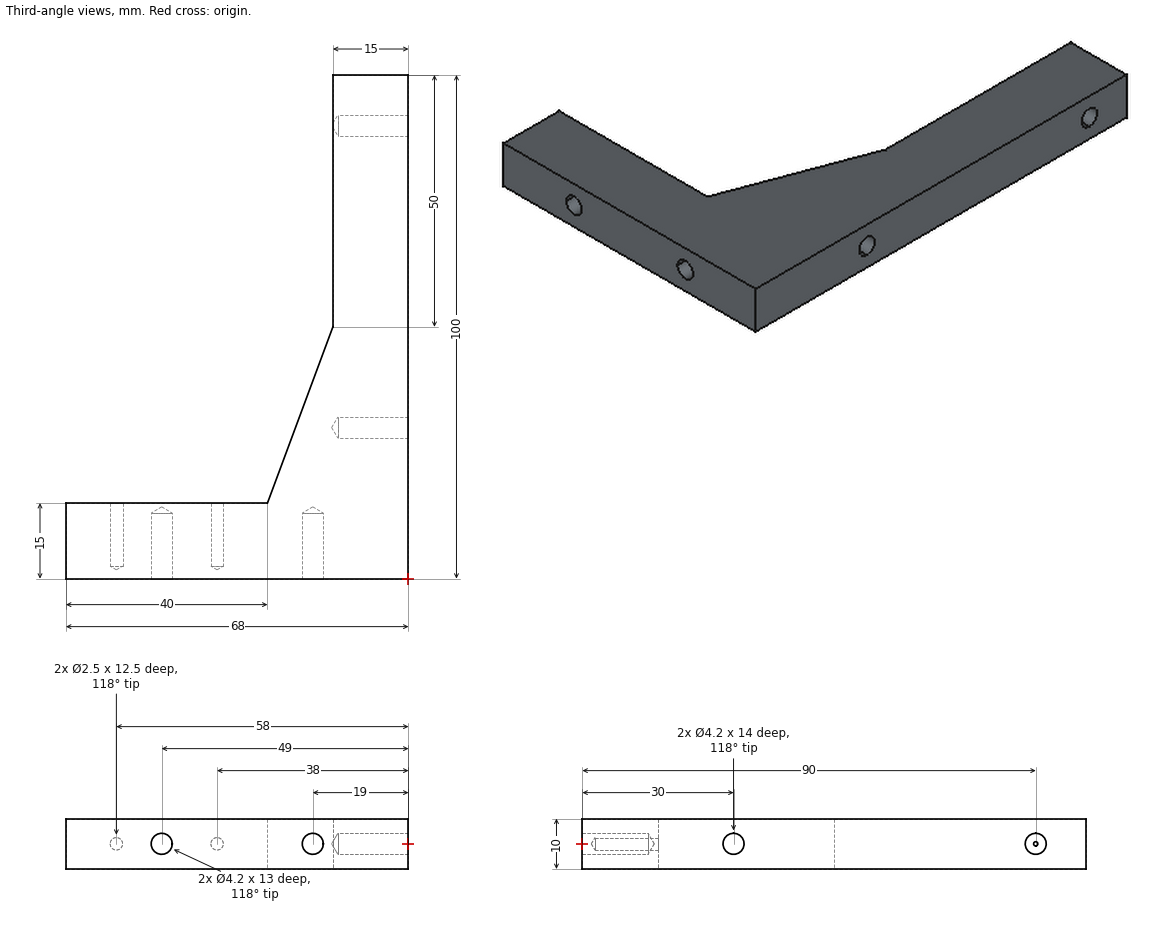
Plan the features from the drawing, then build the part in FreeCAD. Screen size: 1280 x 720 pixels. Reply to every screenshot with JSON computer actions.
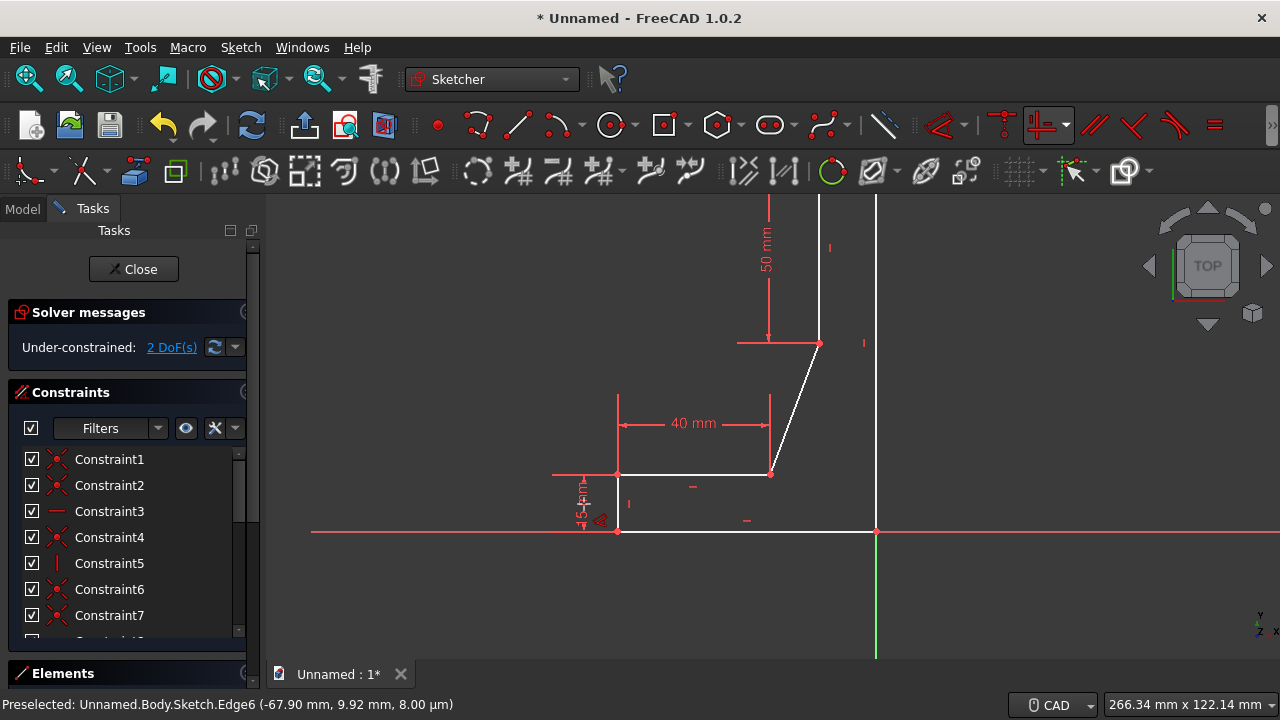
{"action": "left_click", "coordinate": [695, 532]}
{"action": "left_click", "coordinate": [747, 566]}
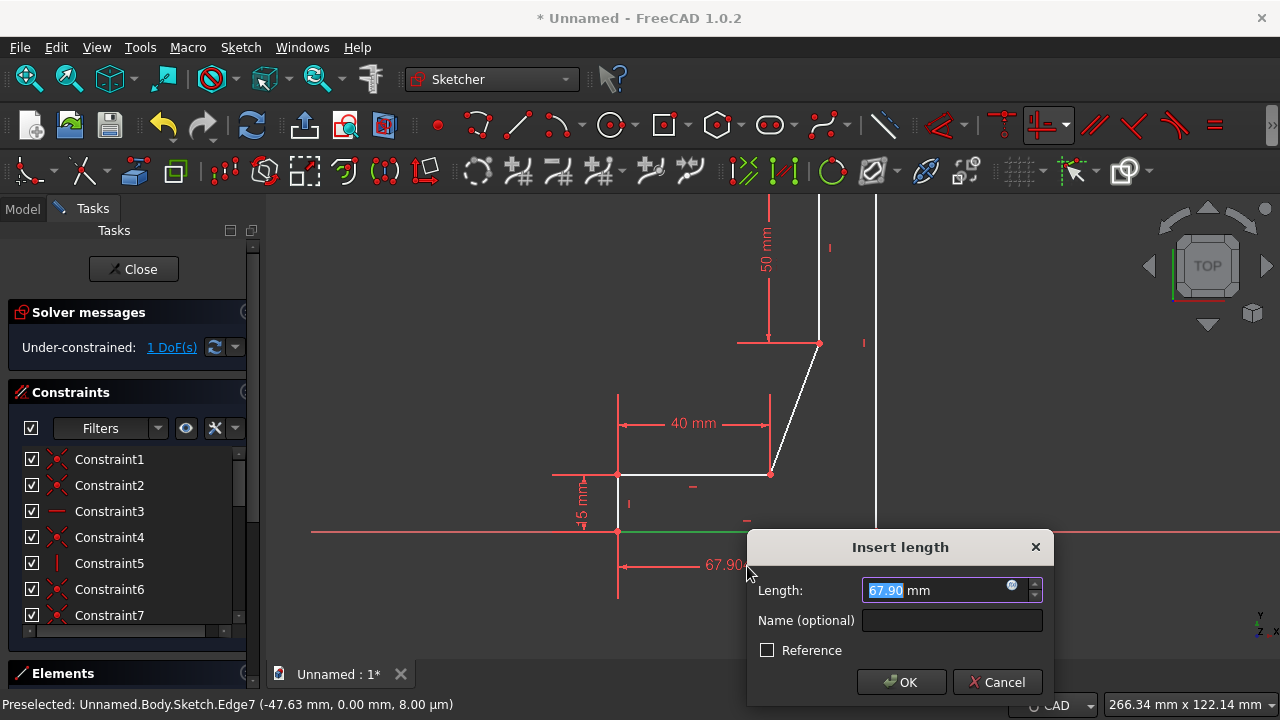
{"action": "type", "text": "68"}
{"action": "key", "text": "Return"}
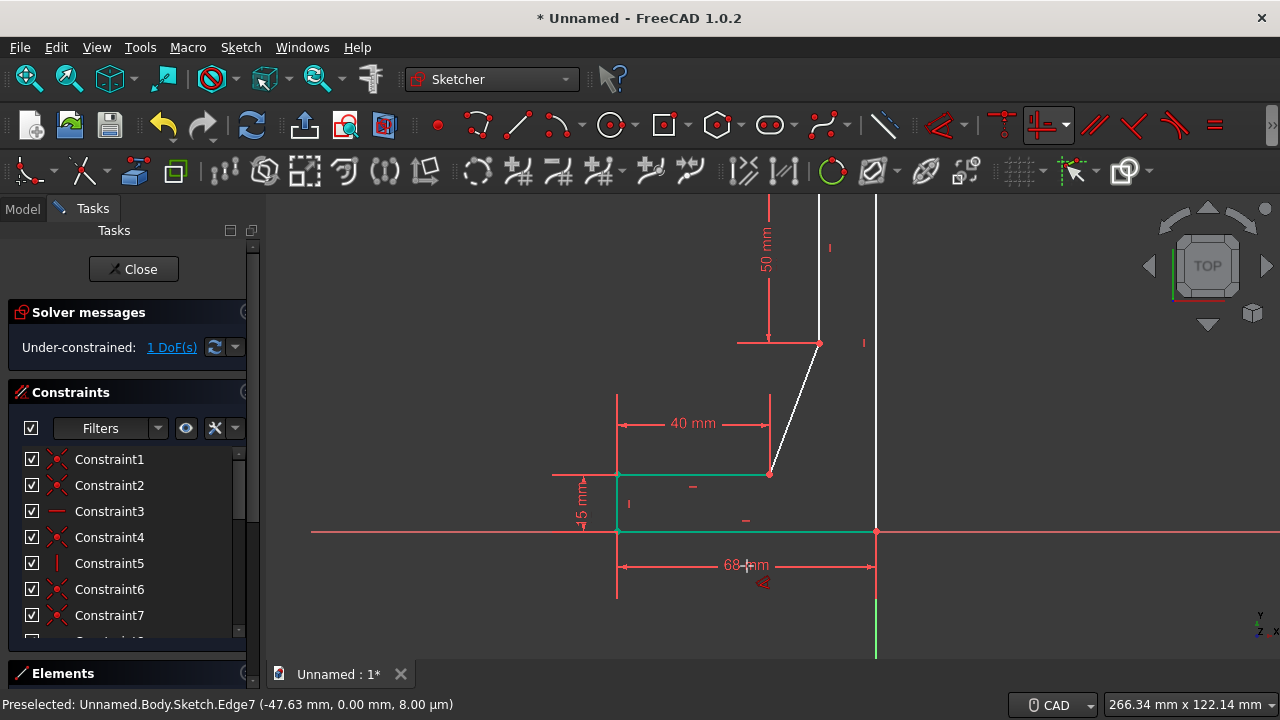
{"action": "left_click", "coordinate": [876, 418]}
{"action": "left_click", "coordinate": [910, 377]}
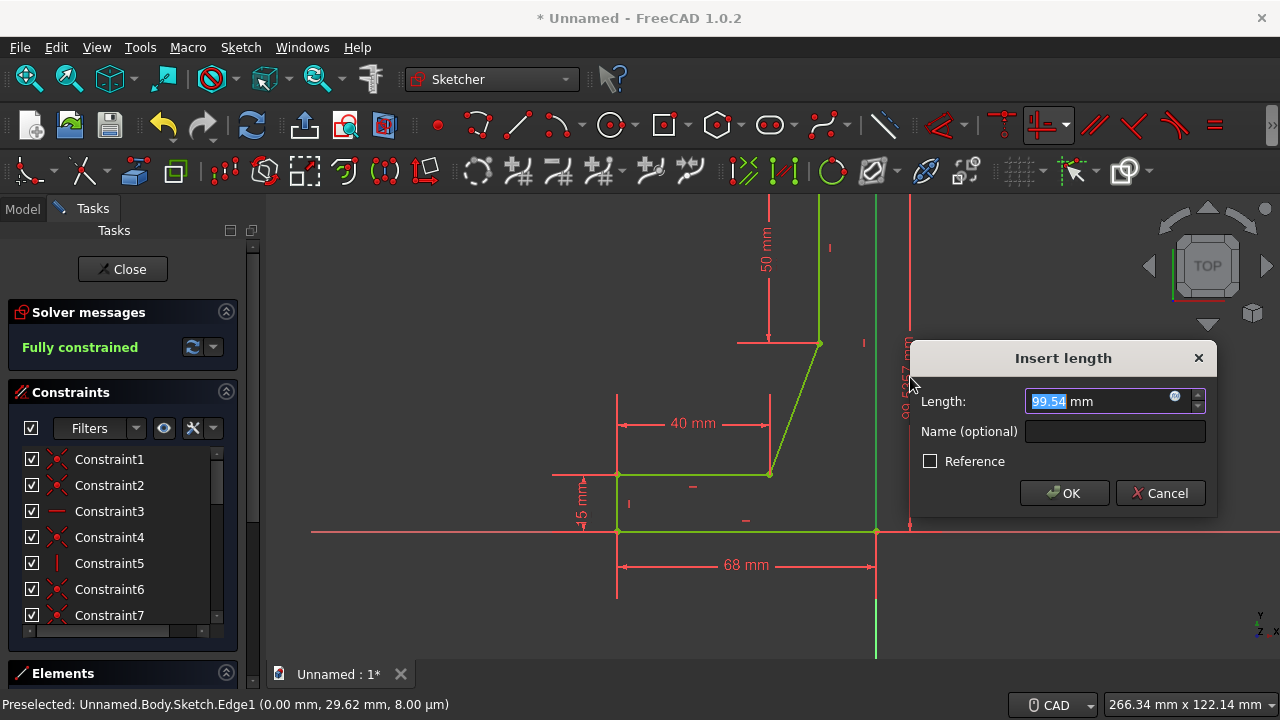
{"action": "type", "text": "100"}
{"action": "key", "text": "Return"}
{"action": "key", "text": "Escape"}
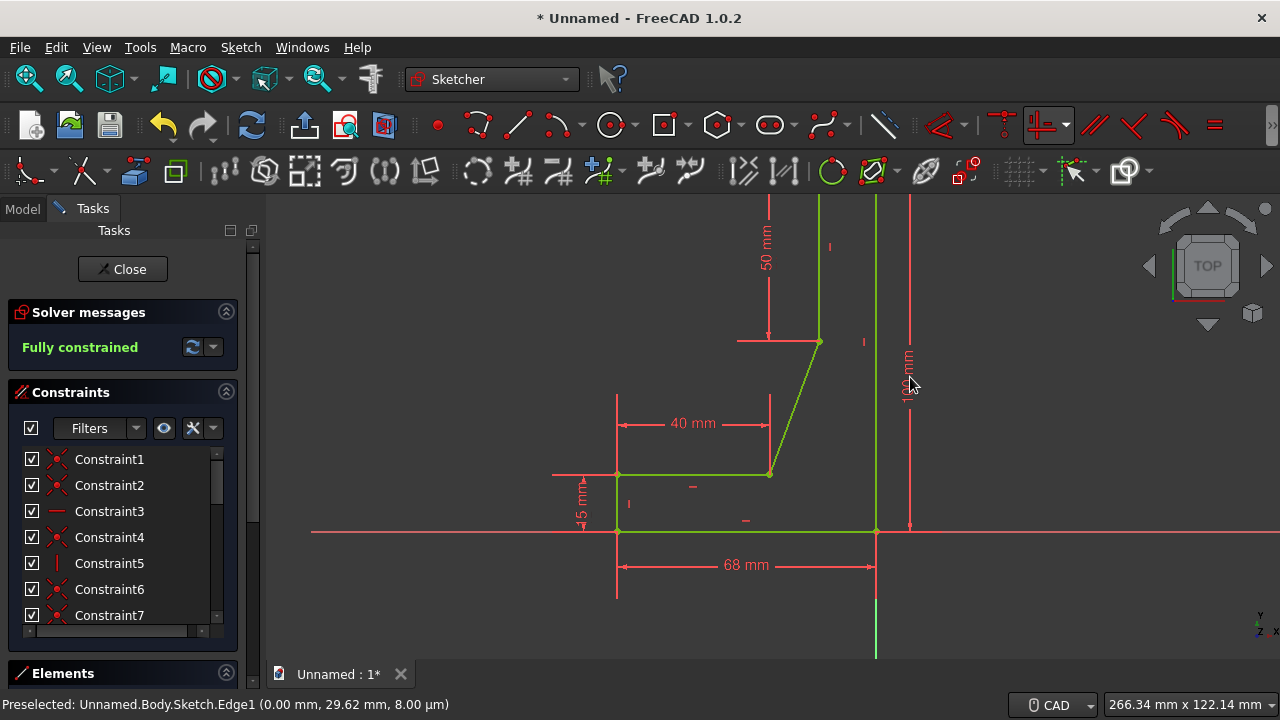
{"action": "left_click", "coordinate": [123, 269]}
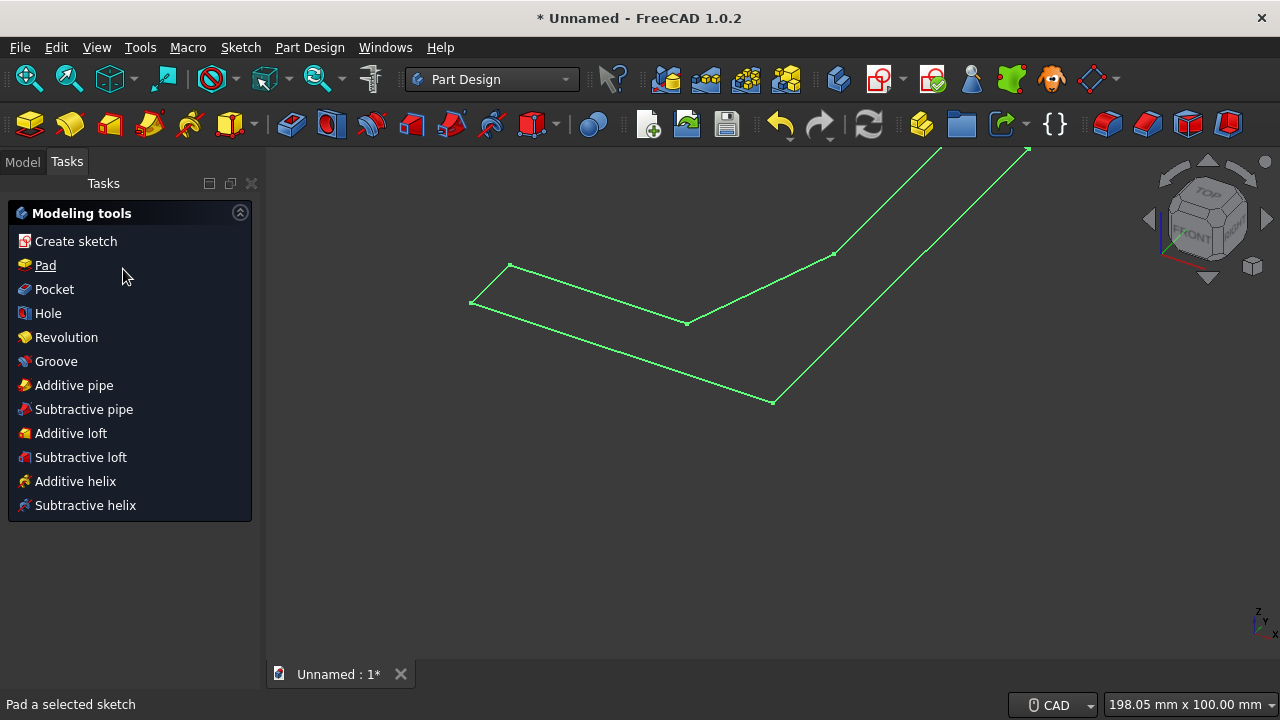
{"action": "left_click", "coordinate": [30, 124]}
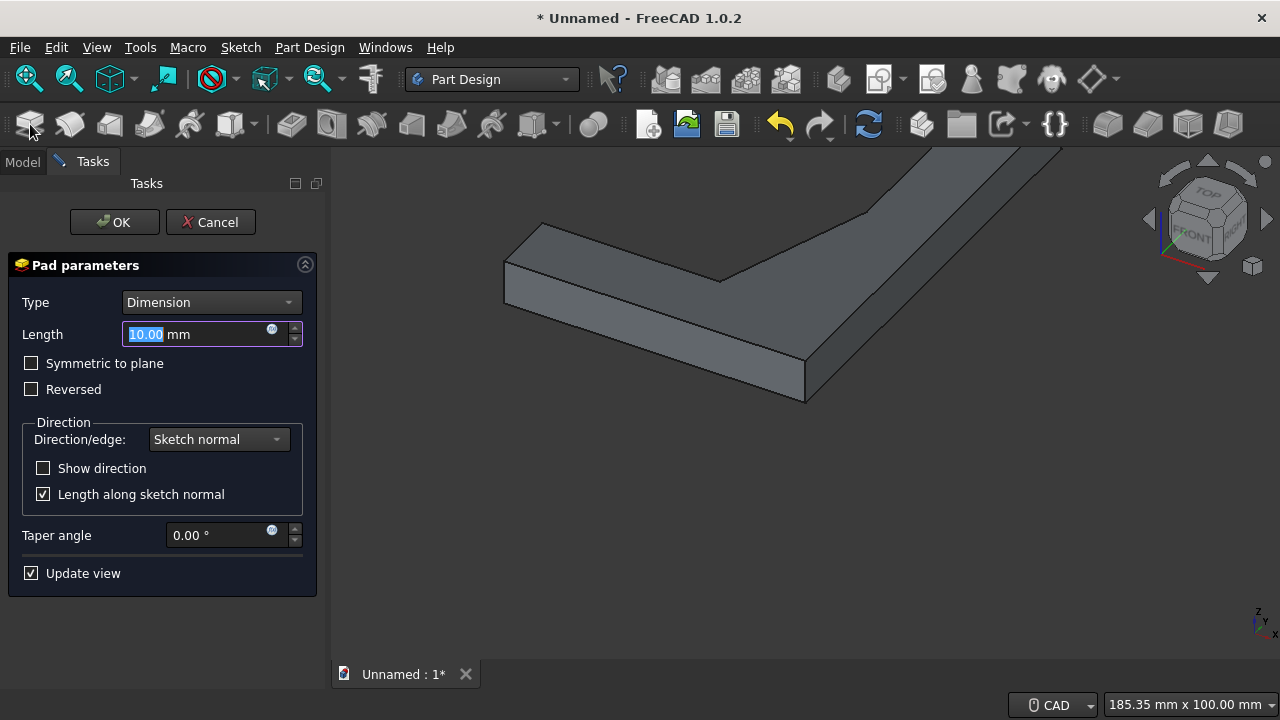
{"action": "type", "text": "10"}
{"action": "key", "text": "Tab"}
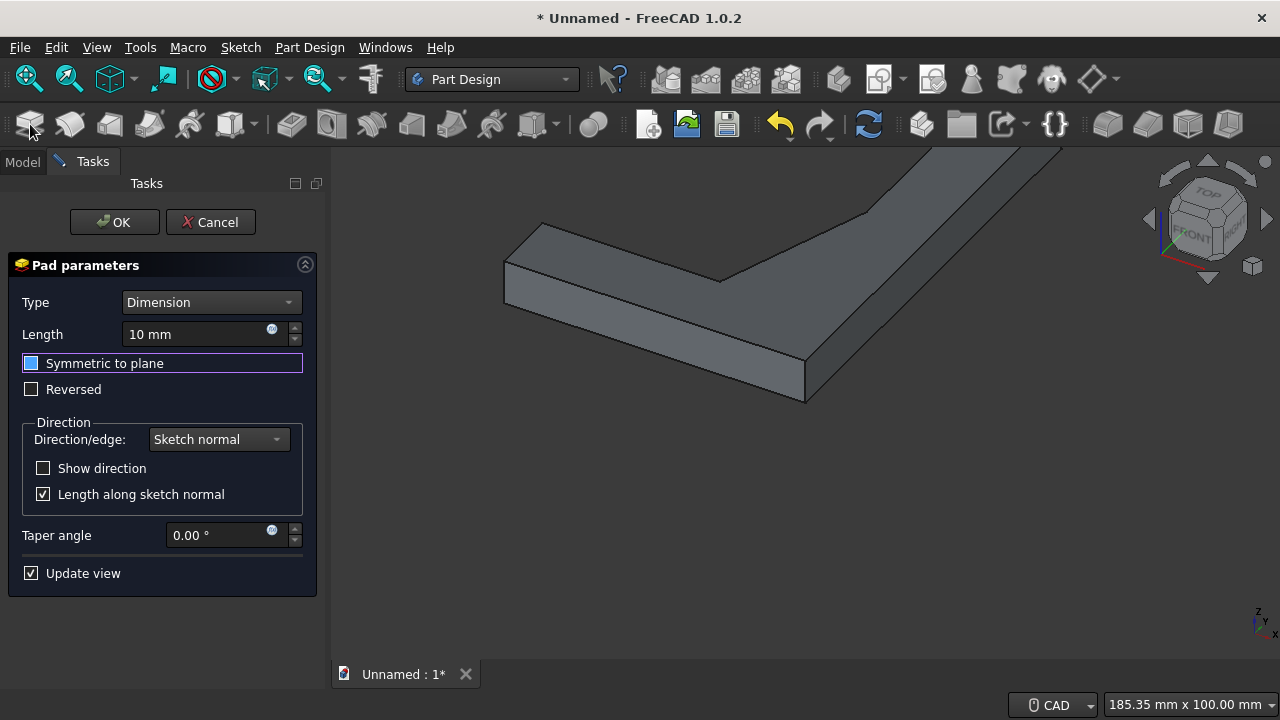
{"action": "left_click", "coordinate": [30, 363]}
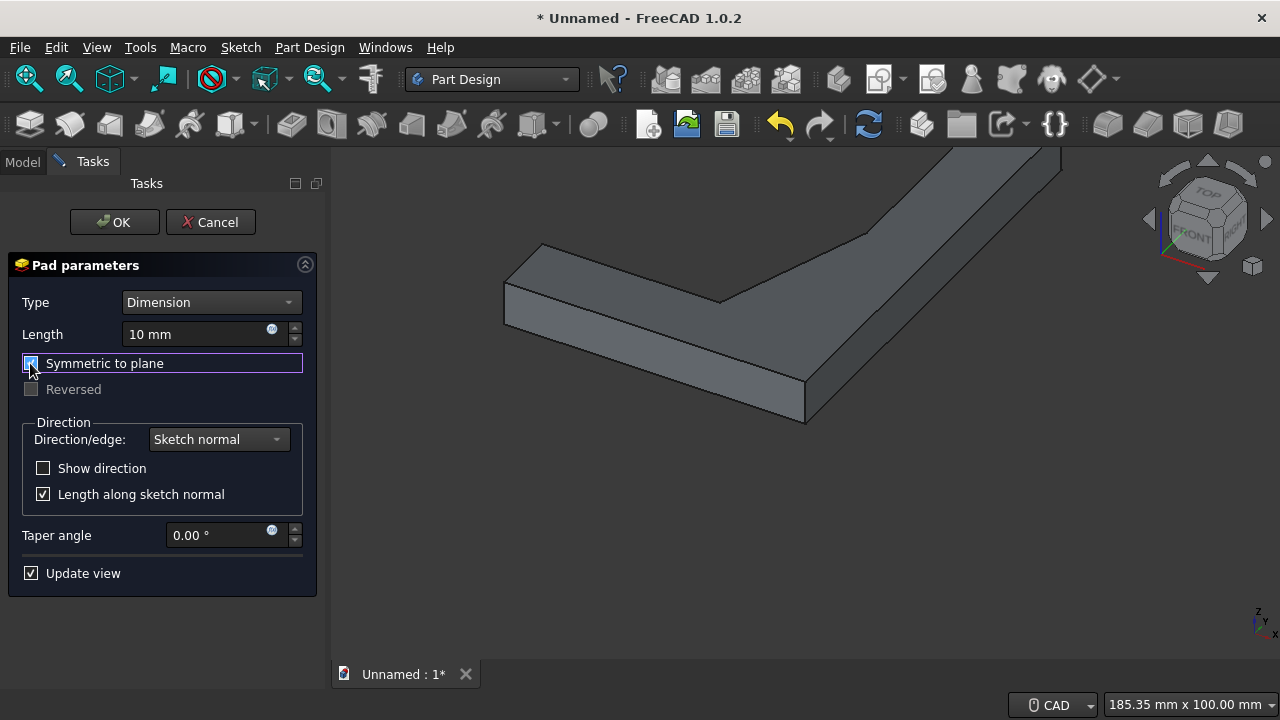
{"action": "left_click", "coordinate": [115, 222]}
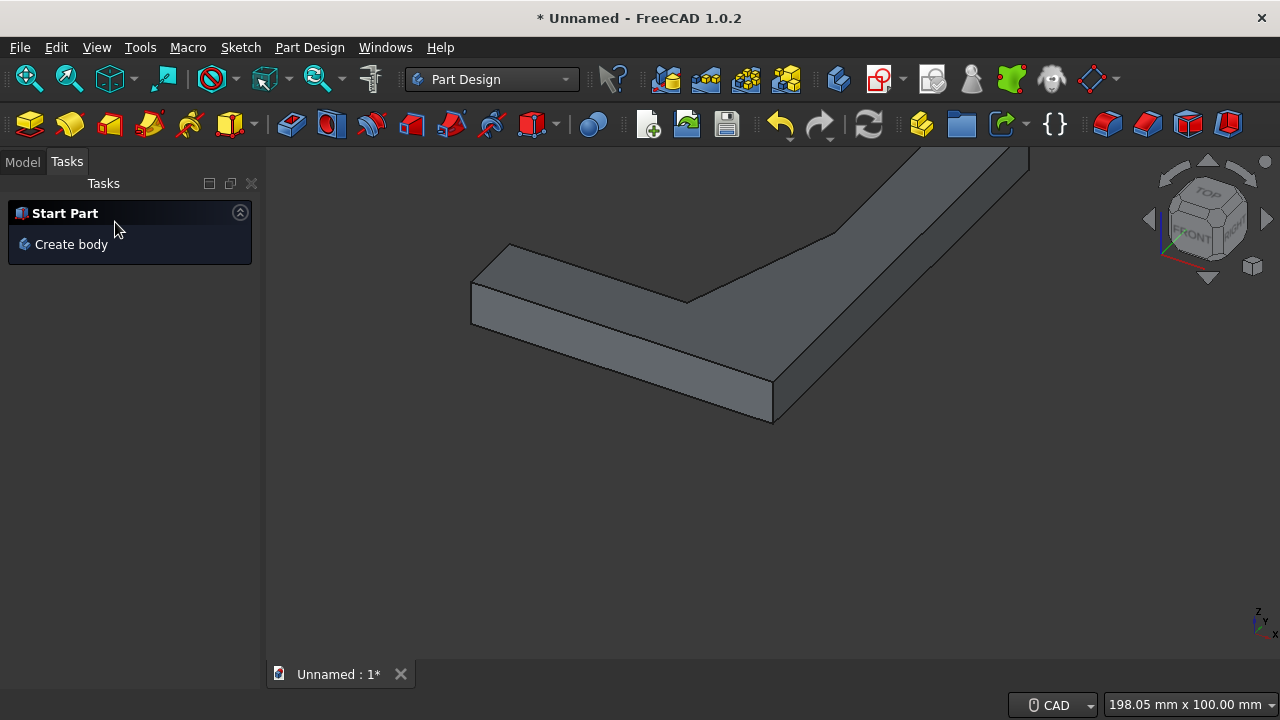
{"action": "left_click", "coordinate": [30, 80]}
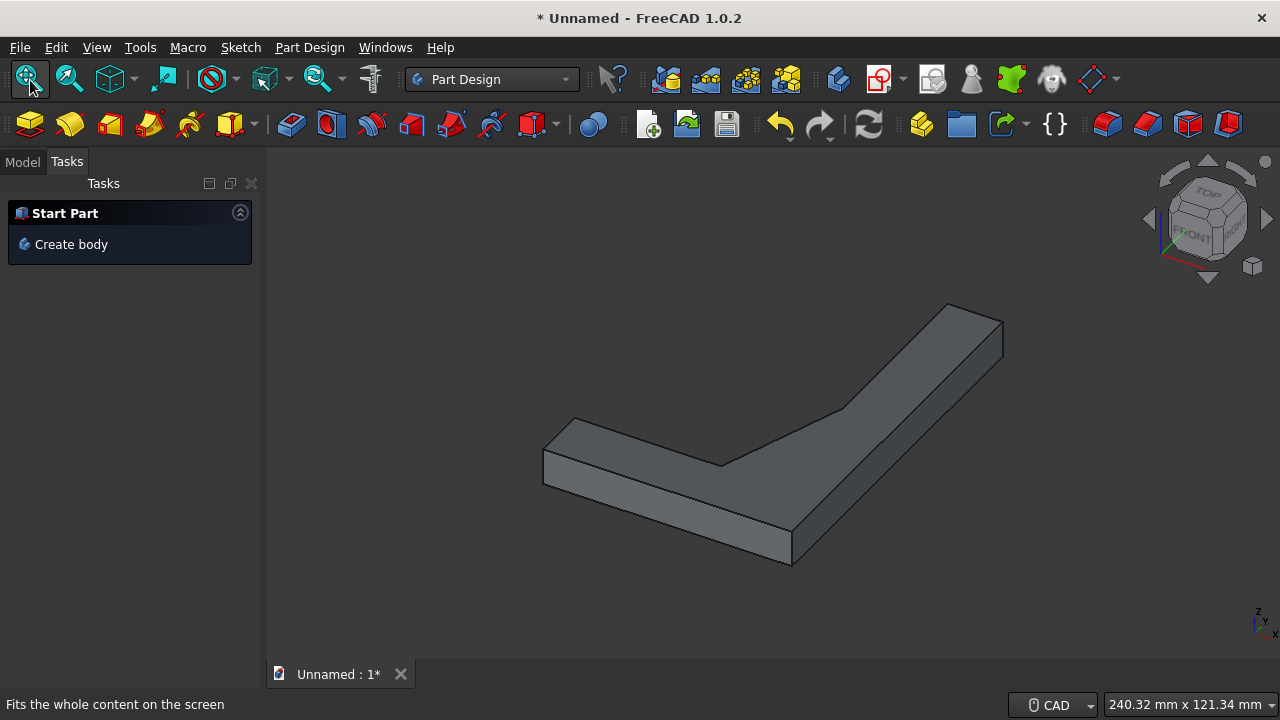
{"action": "left_click", "coordinate": [880, 80]}